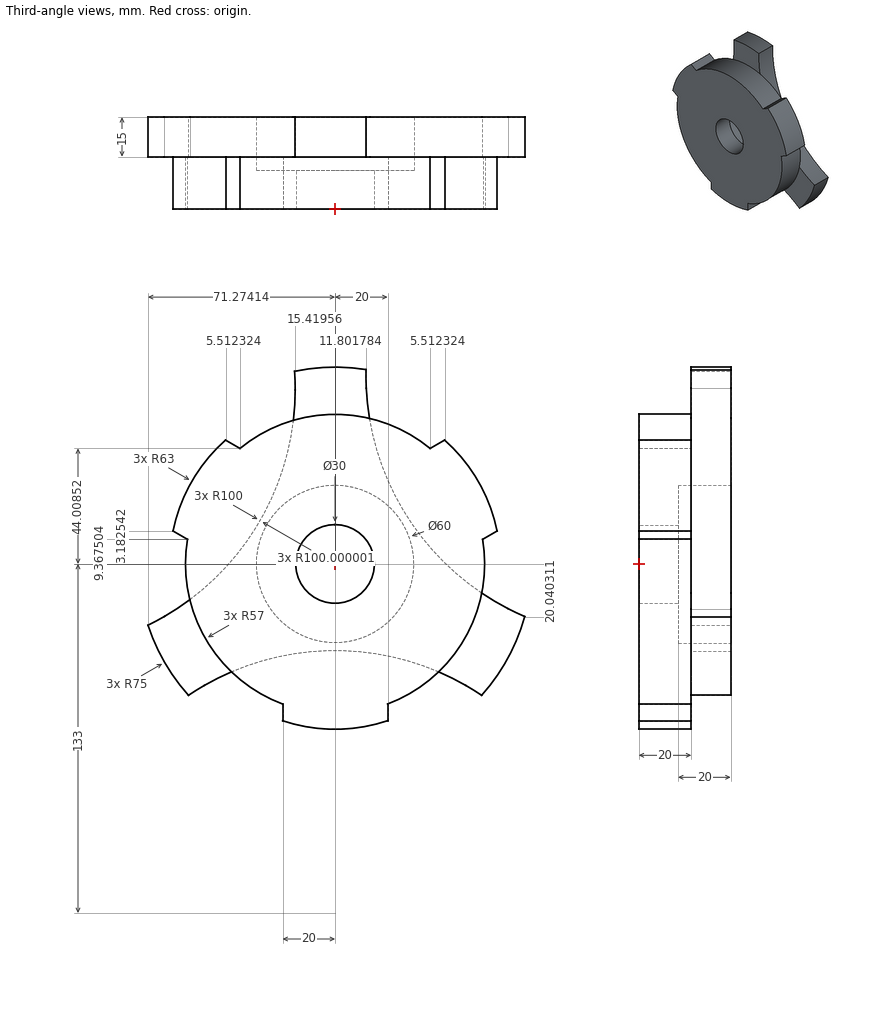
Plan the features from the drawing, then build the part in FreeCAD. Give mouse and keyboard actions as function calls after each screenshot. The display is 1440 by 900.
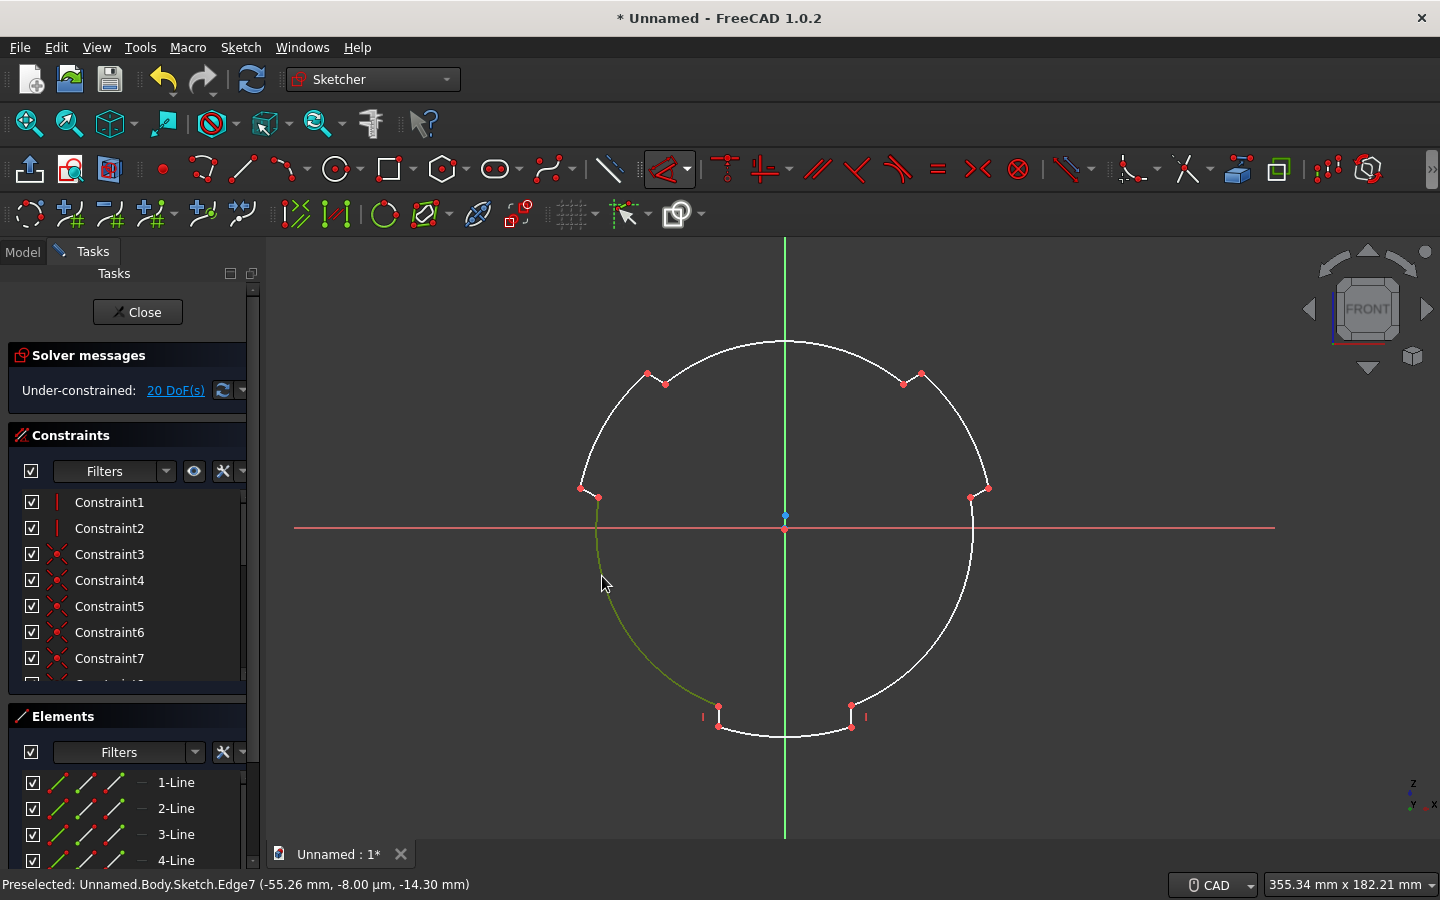
click(758, 735)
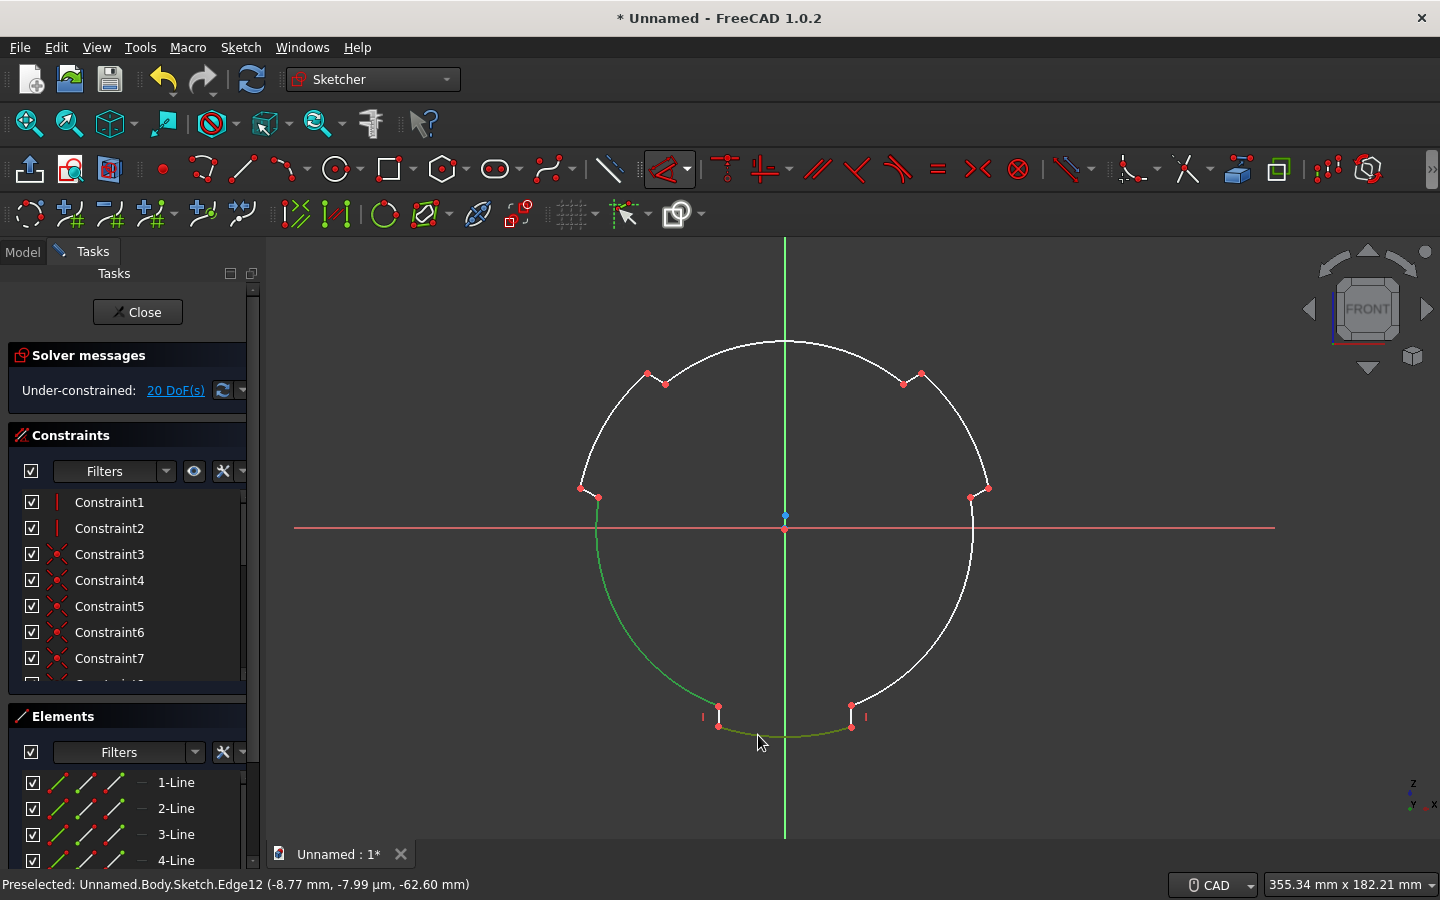
click(726, 170)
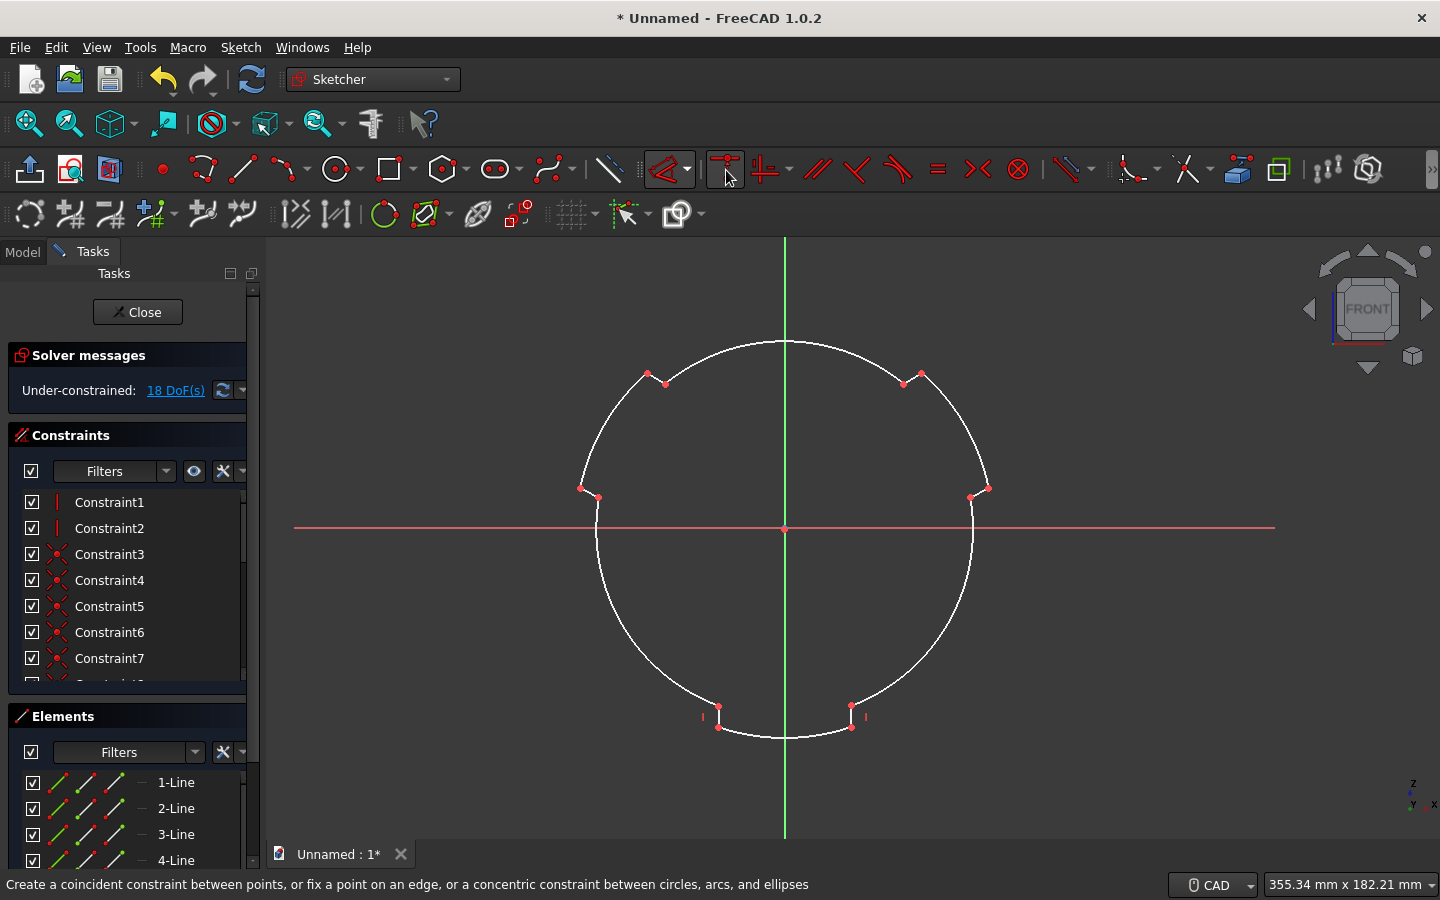
drag(774, 518, 795, 540)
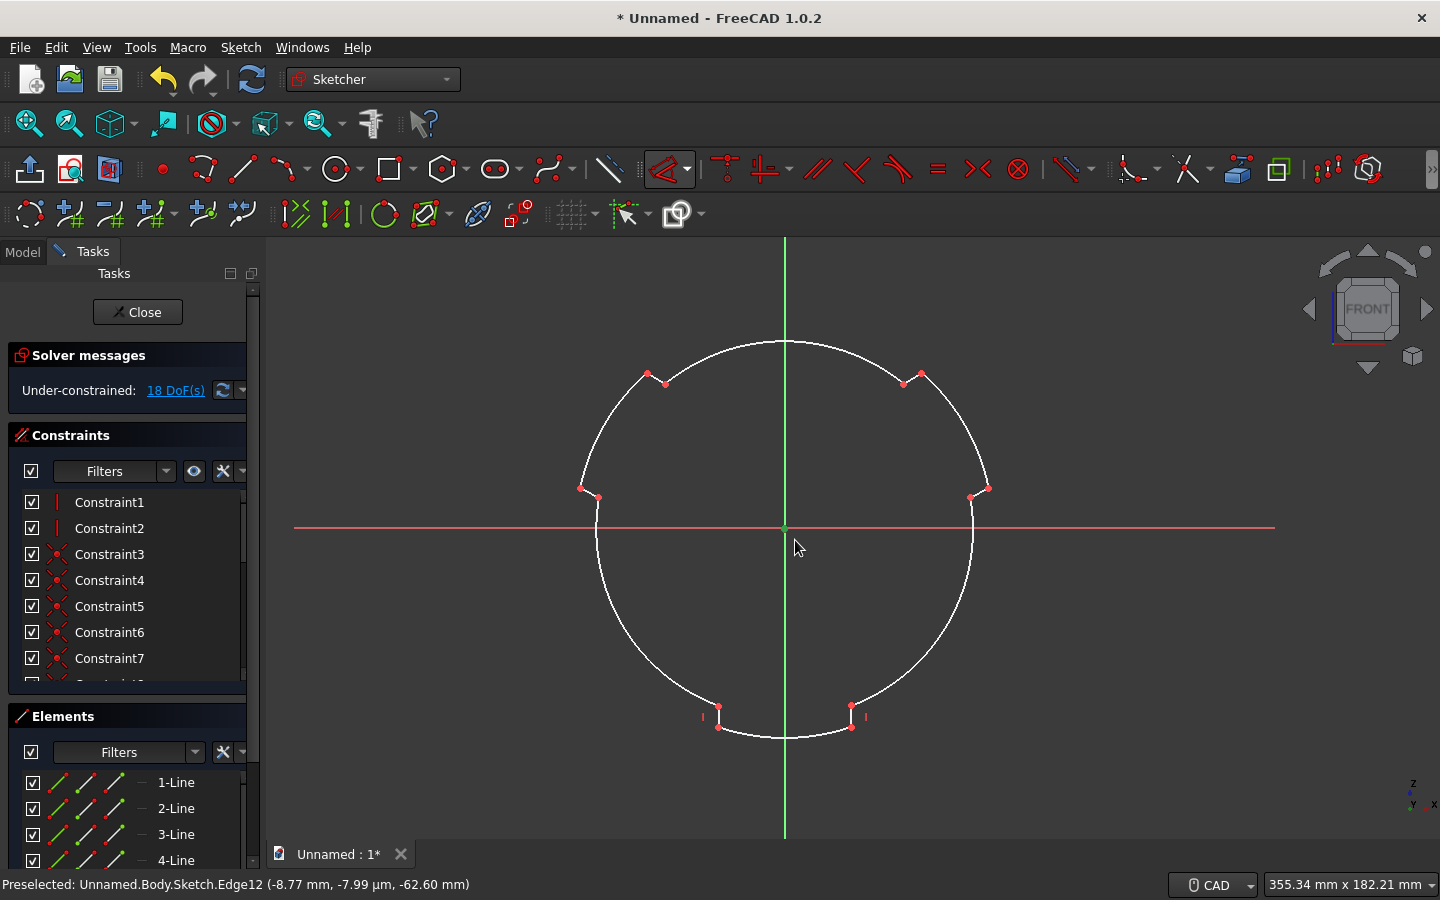
click(726, 170)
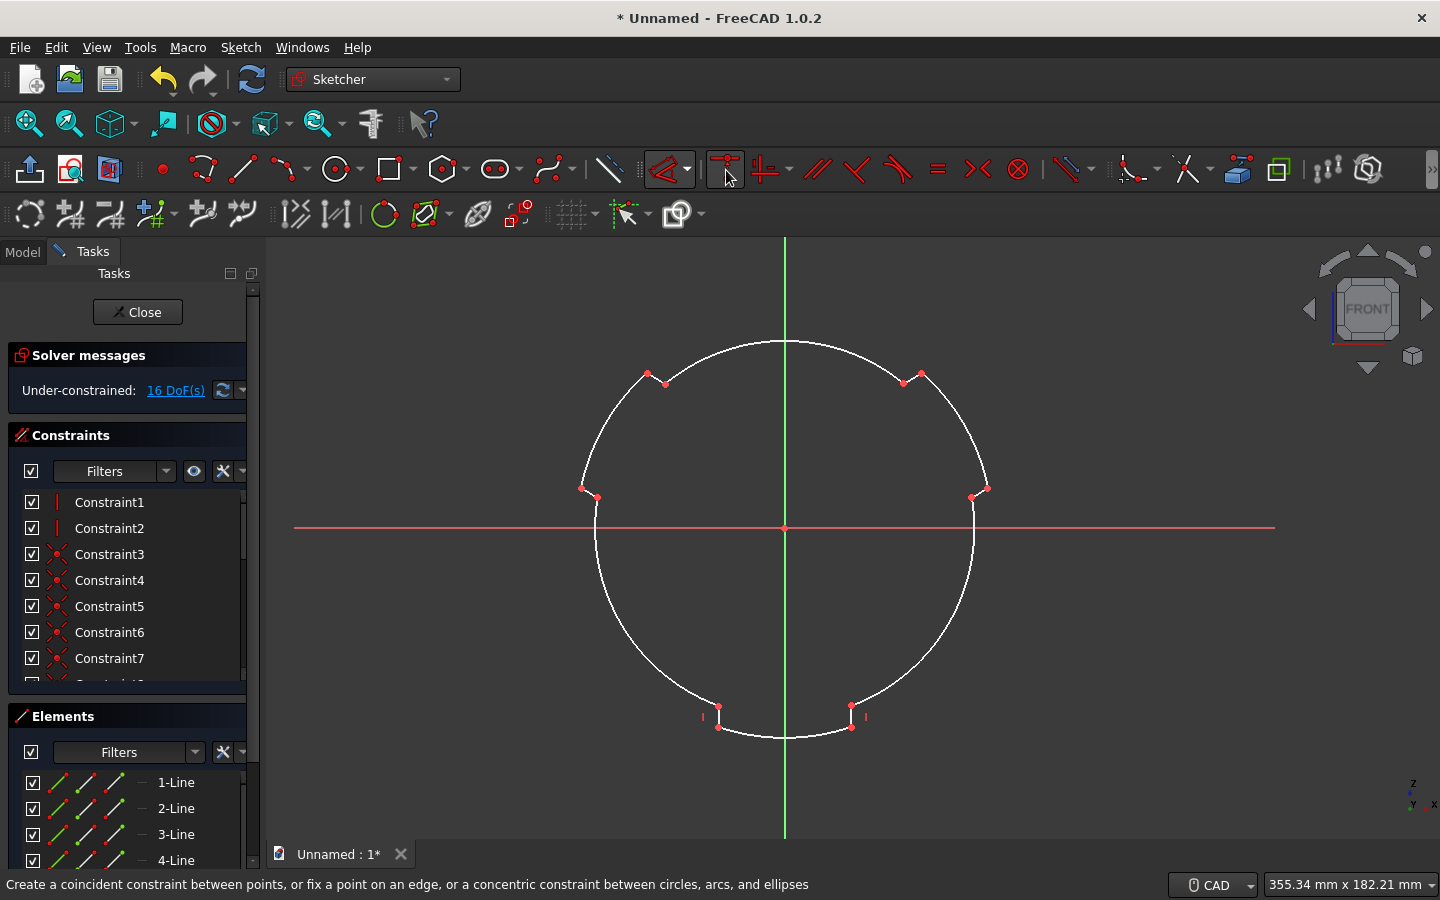
click(601, 576)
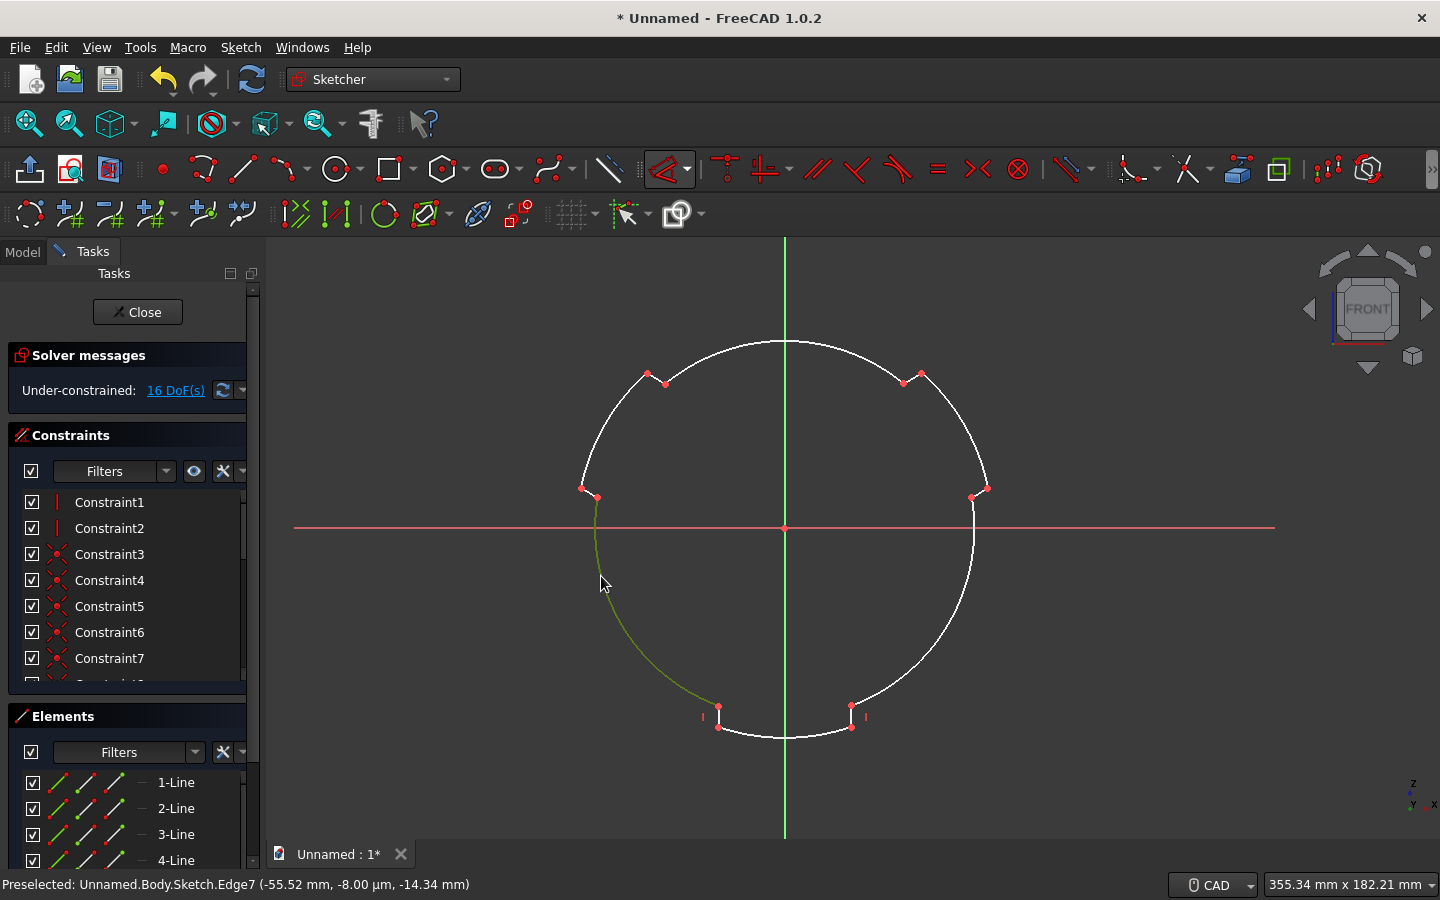
click(836, 348)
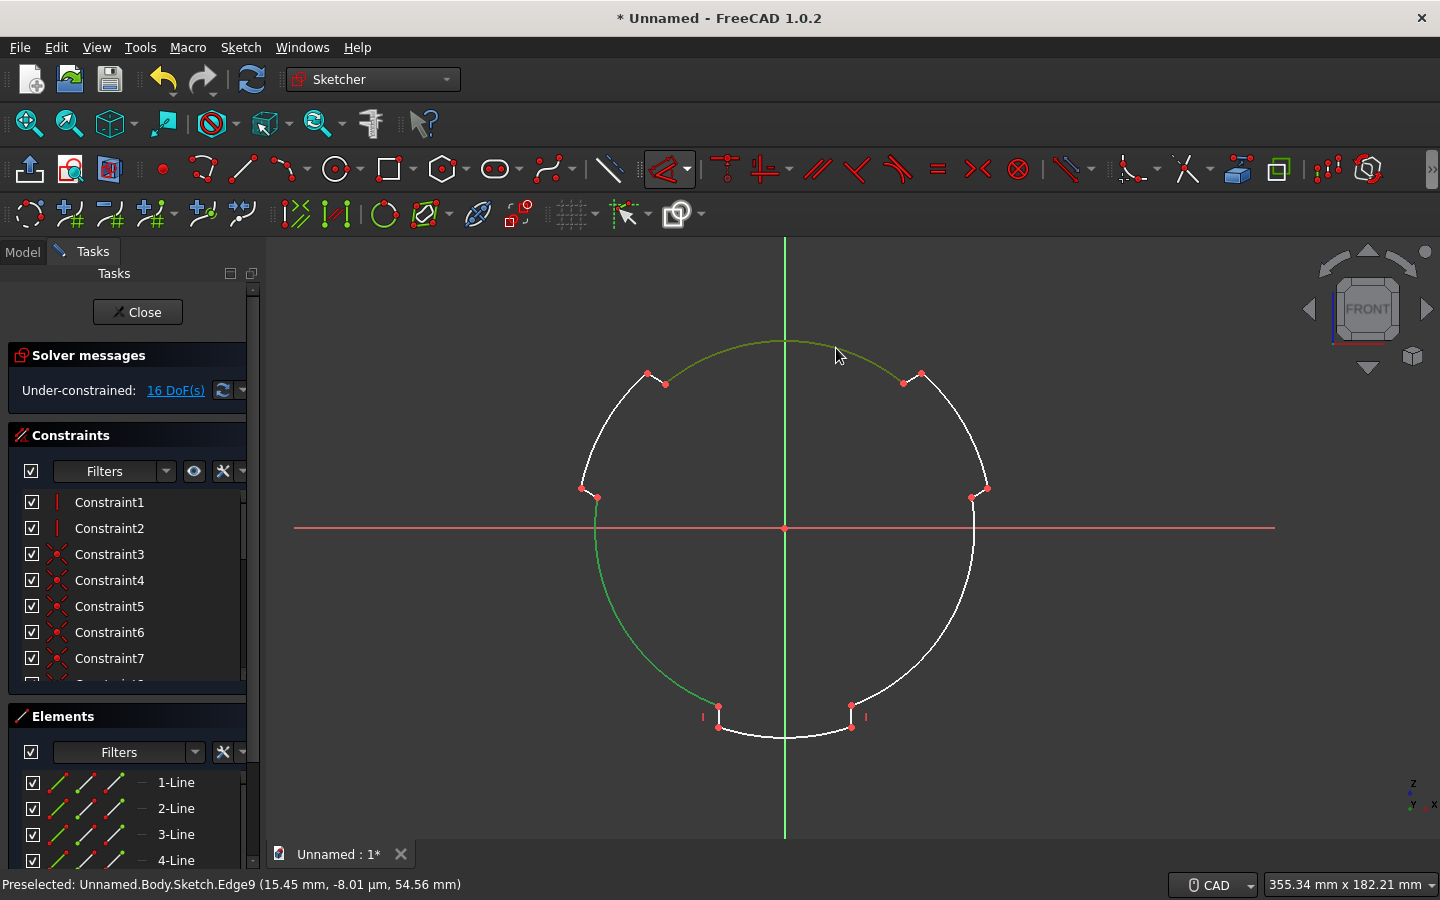
click(917, 665)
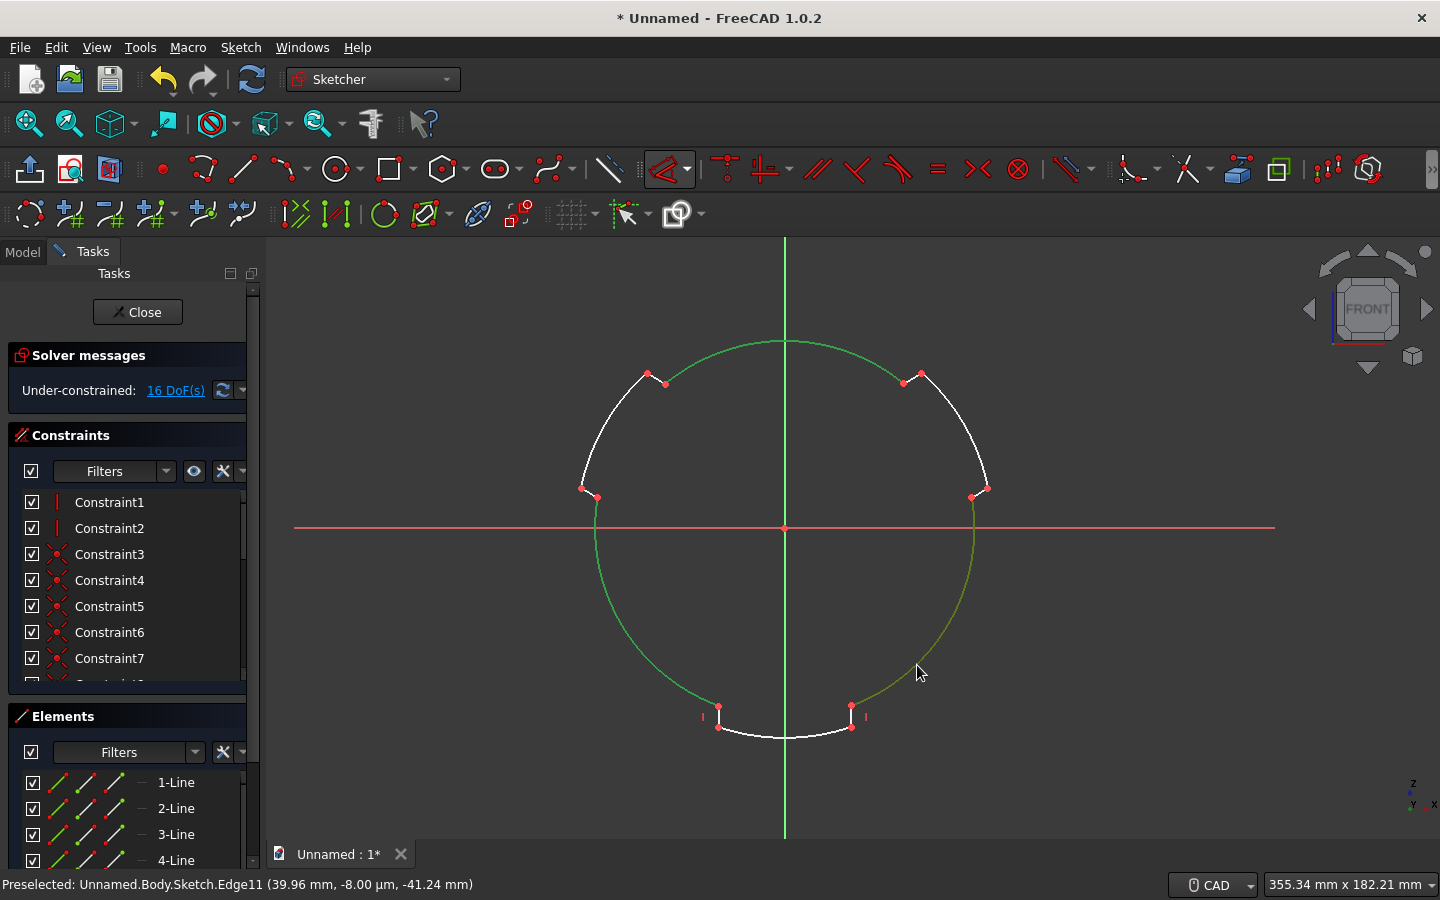
click(938, 170)